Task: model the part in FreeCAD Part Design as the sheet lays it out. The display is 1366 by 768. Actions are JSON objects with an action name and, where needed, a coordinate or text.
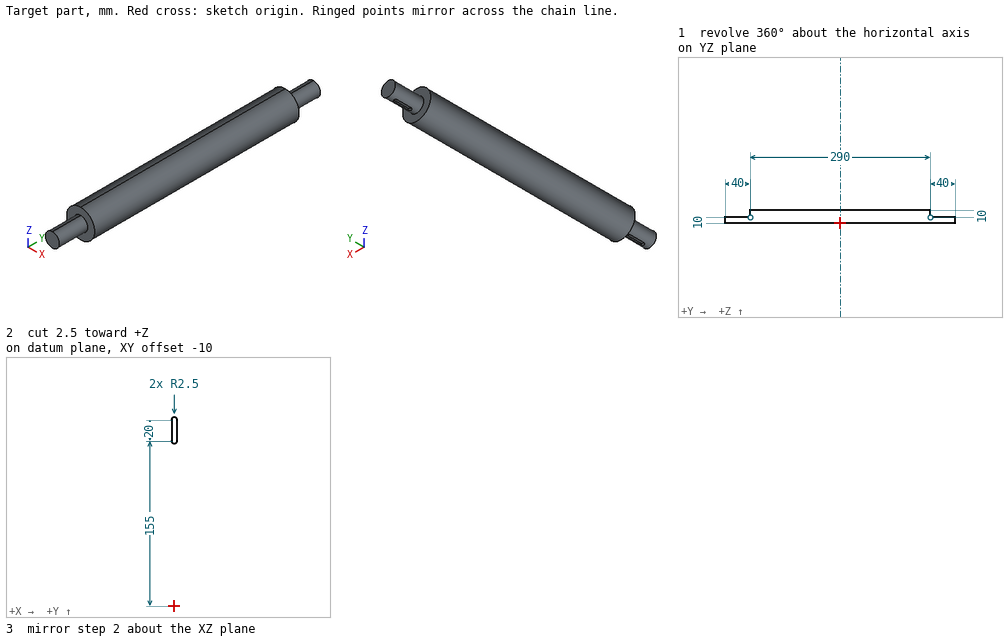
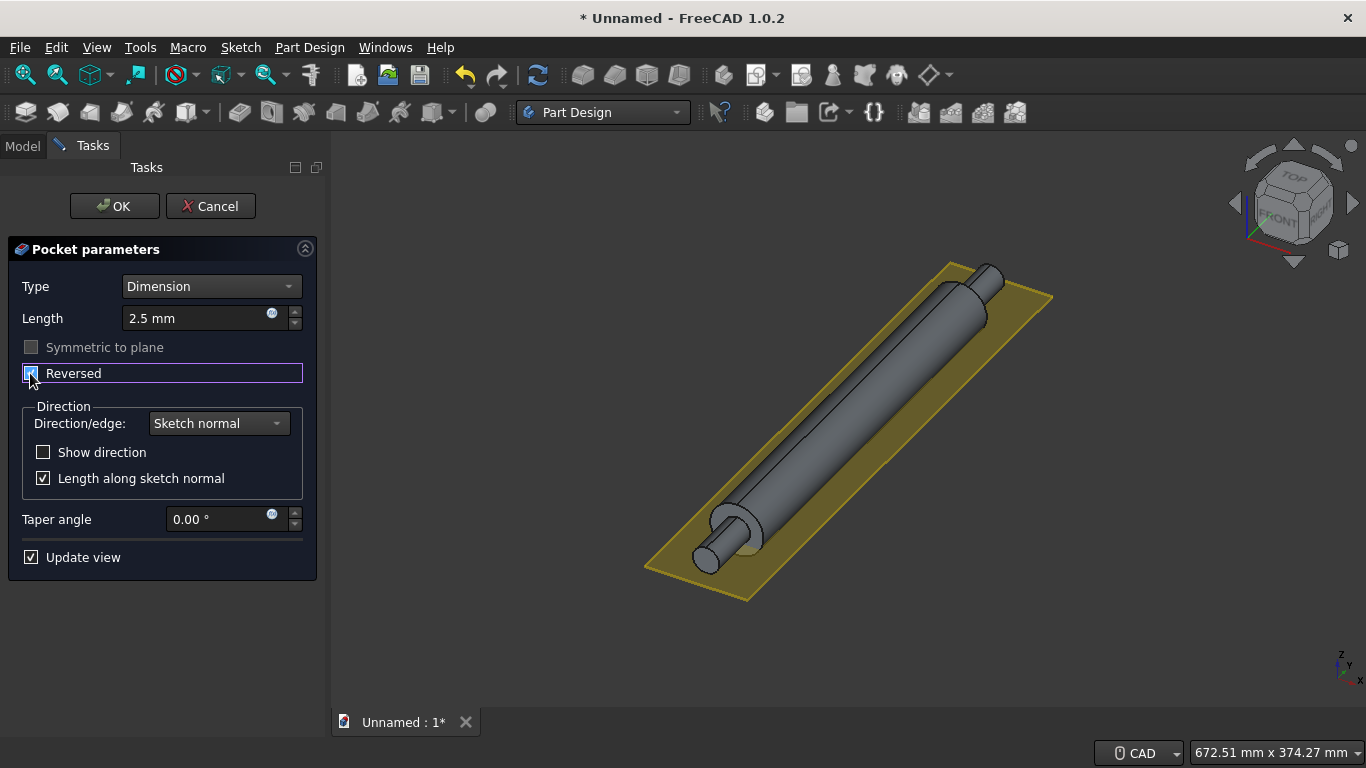
{"action": "left_click", "coordinate": [115, 206]}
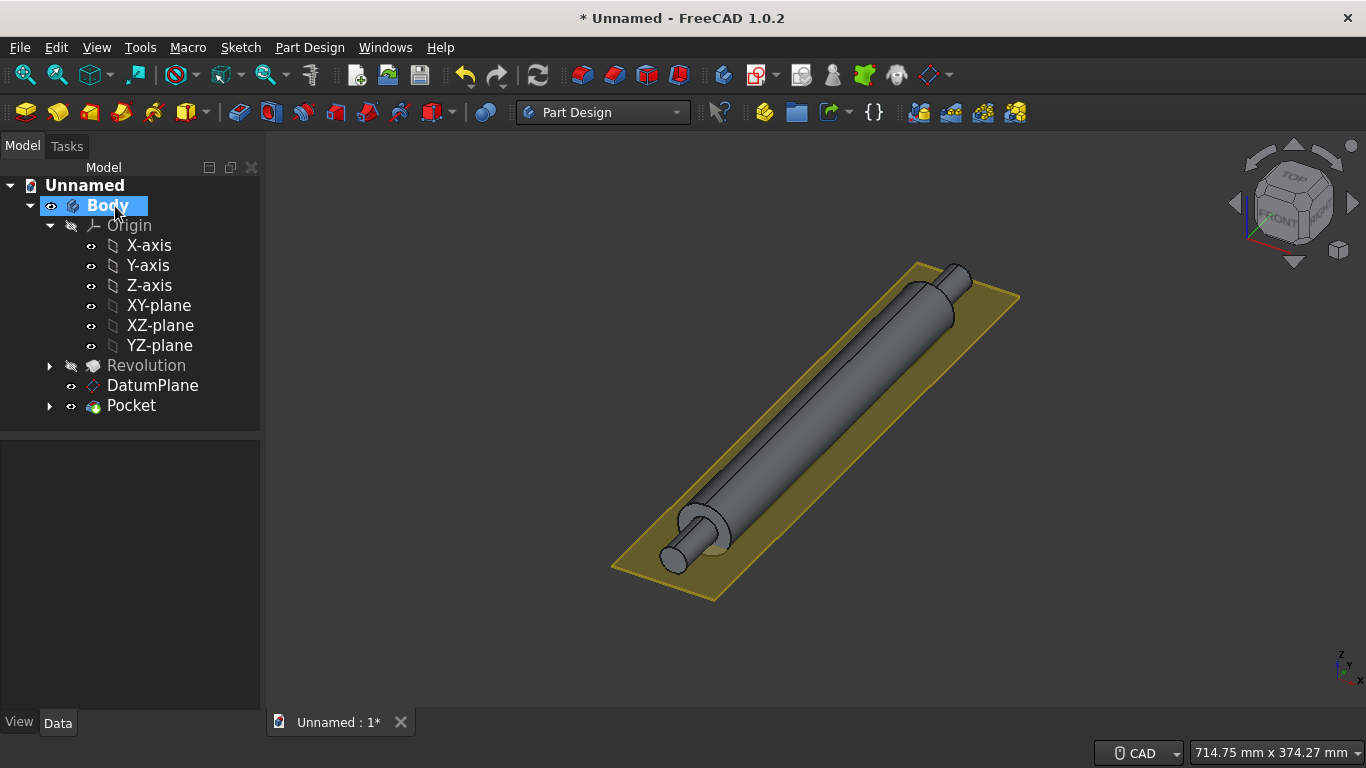
{"action": "left_click", "coordinate": [116, 386]}
{"action": "key", "text": "space"}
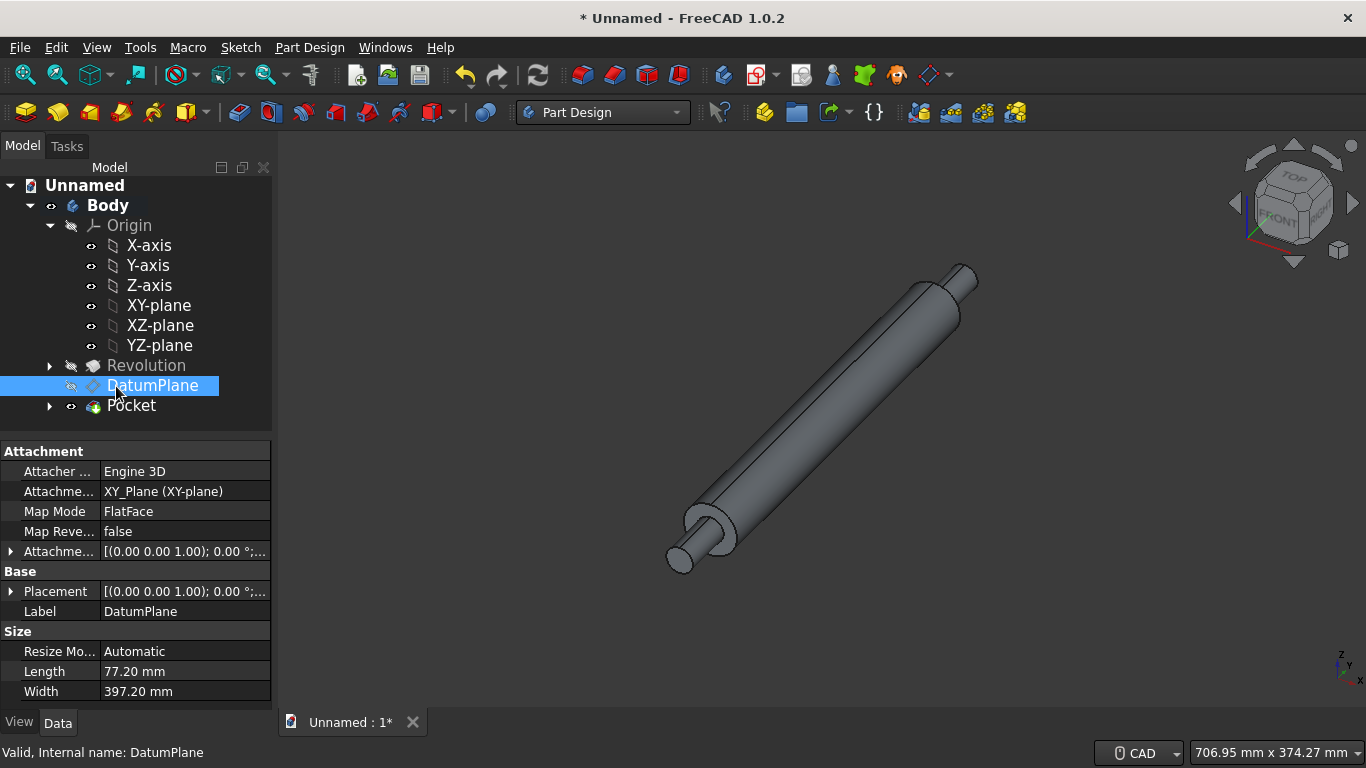
{"action": "left_click", "coordinate": [116, 406]}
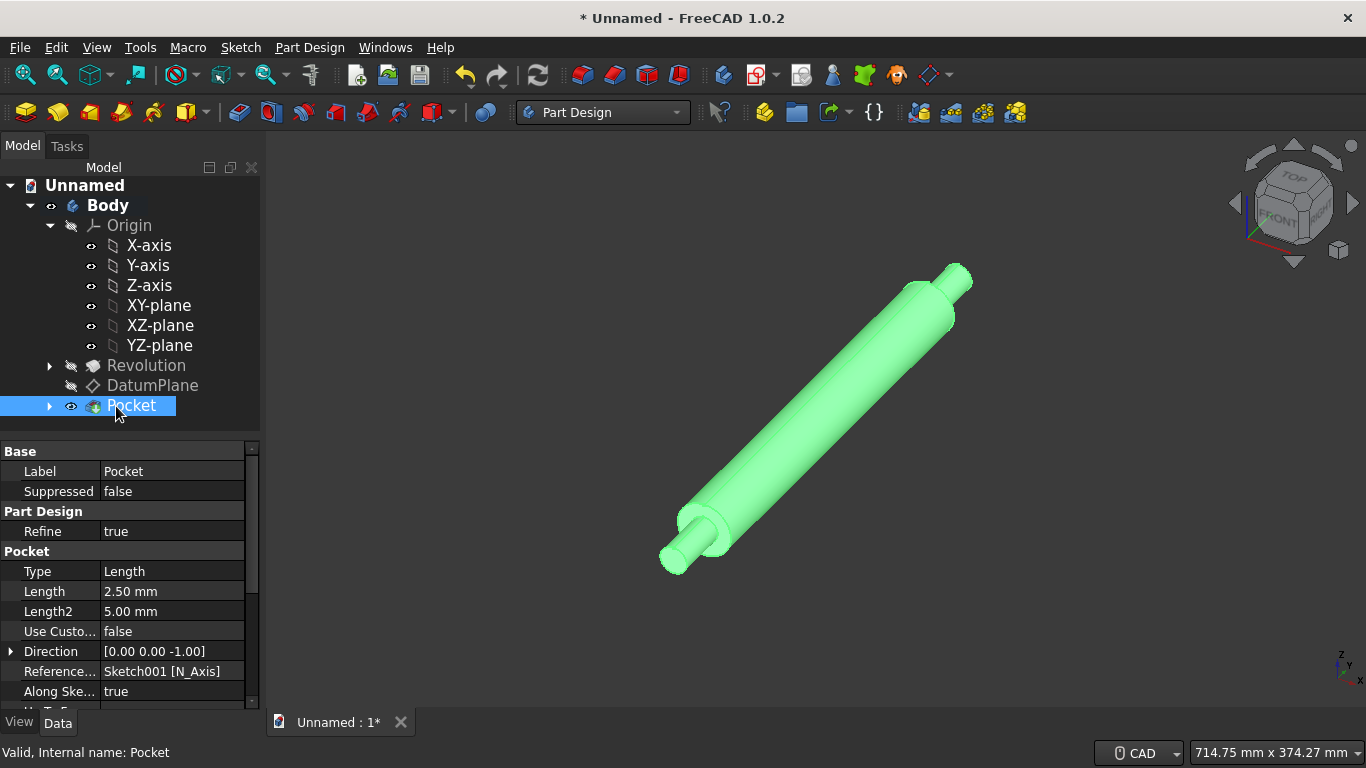
{"action": "left_click", "coordinate": [920, 112]}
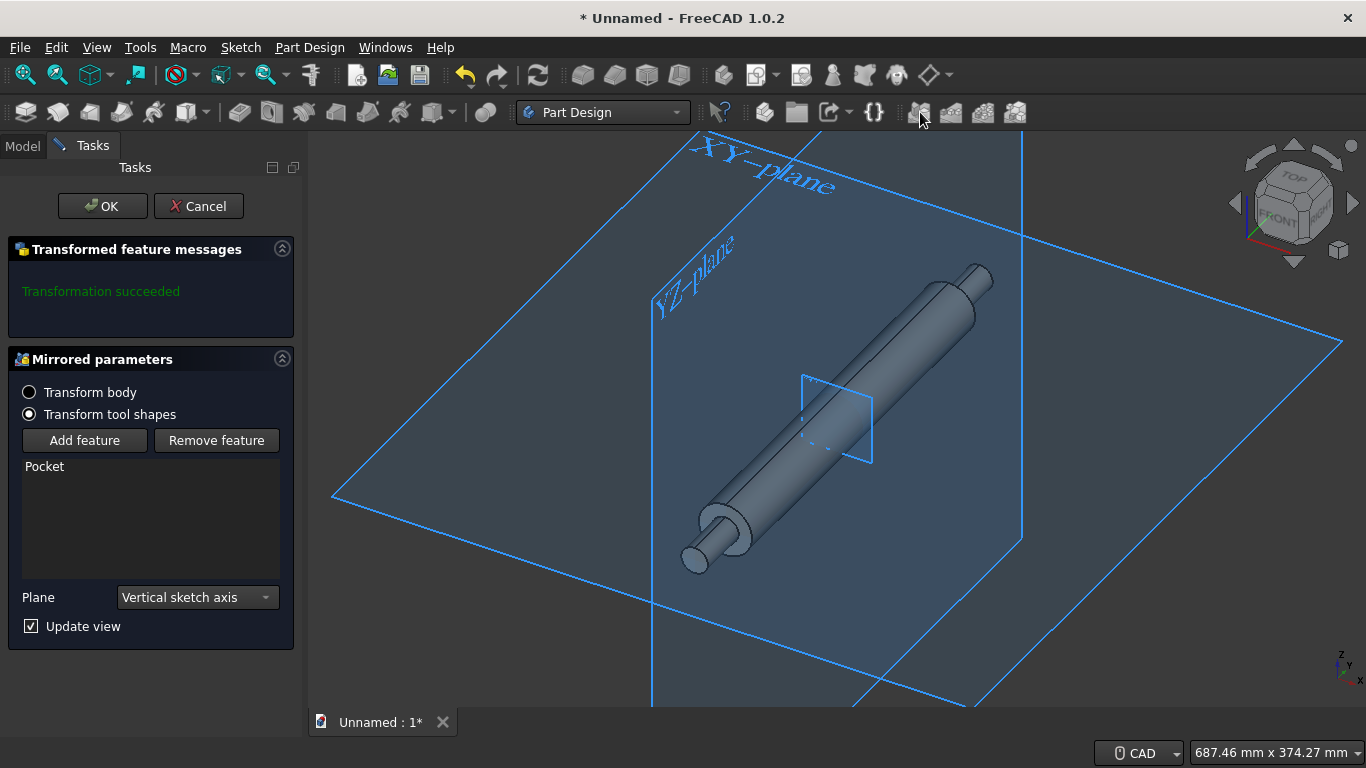
{"action": "left_click", "coordinate": [198, 598]}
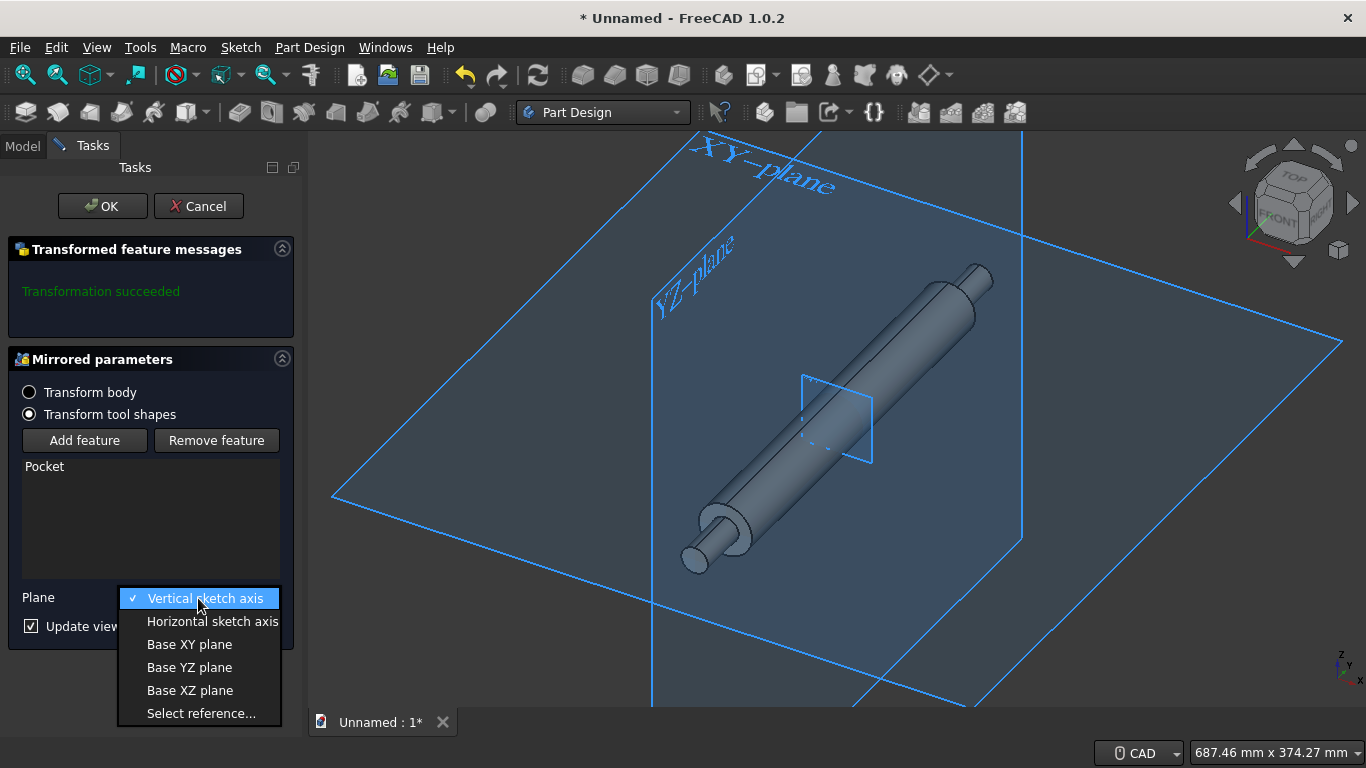
{"action": "left_click", "coordinate": [198, 690]}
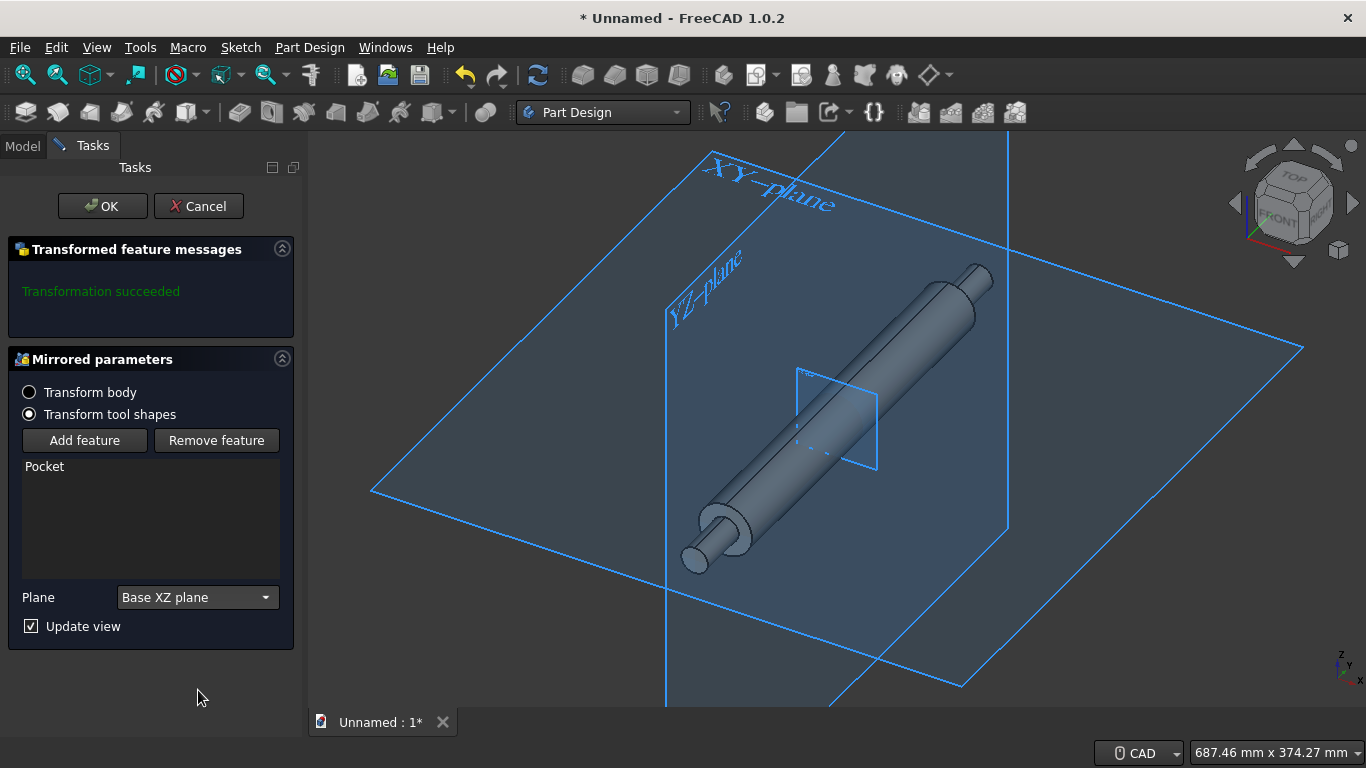
{"action": "left_click", "coordinate": [103, 206]}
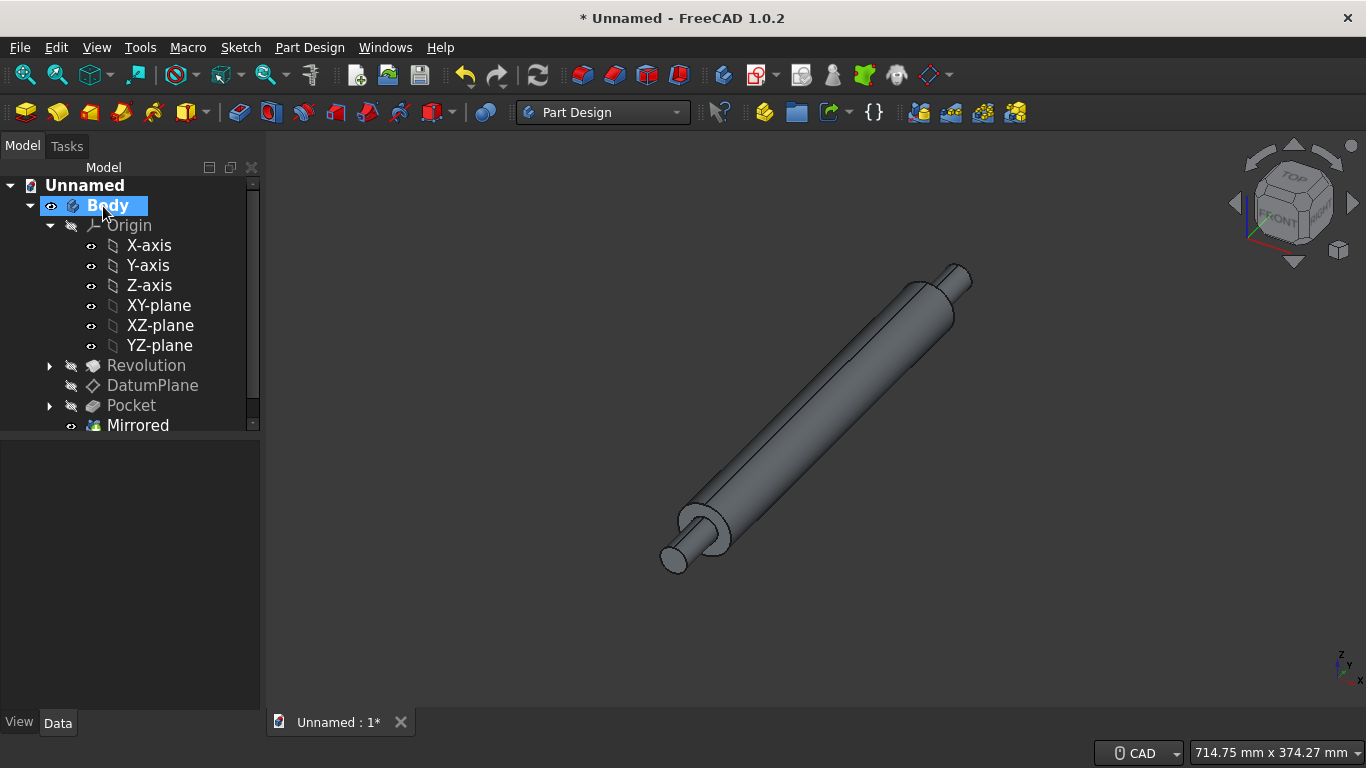
{"action": "key", "text": "0"}